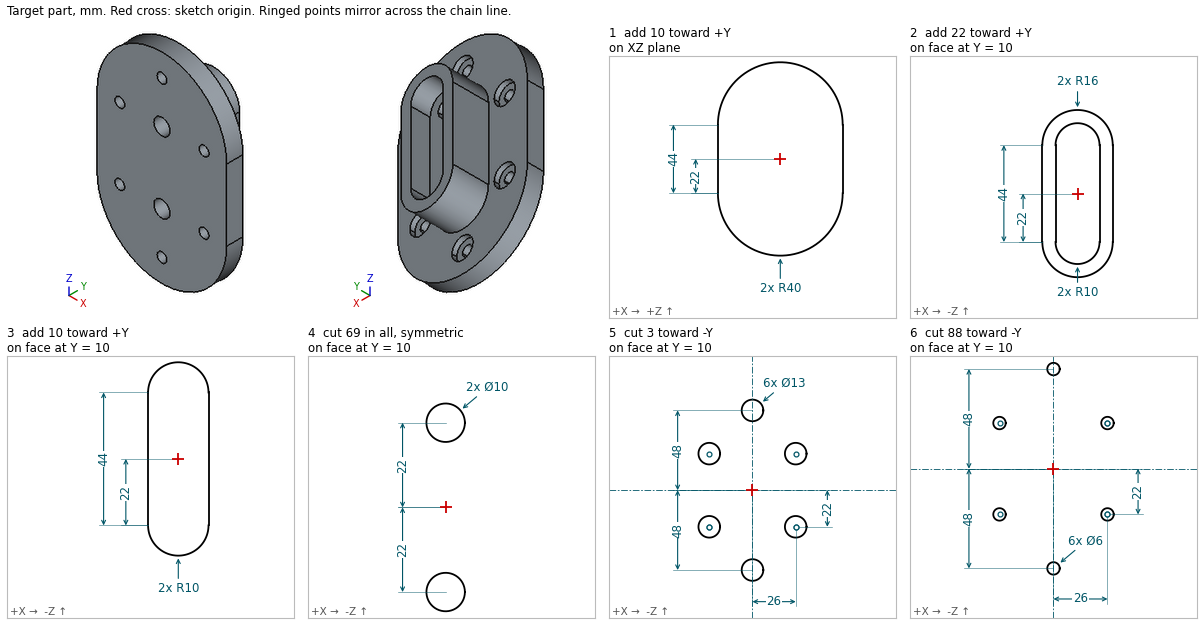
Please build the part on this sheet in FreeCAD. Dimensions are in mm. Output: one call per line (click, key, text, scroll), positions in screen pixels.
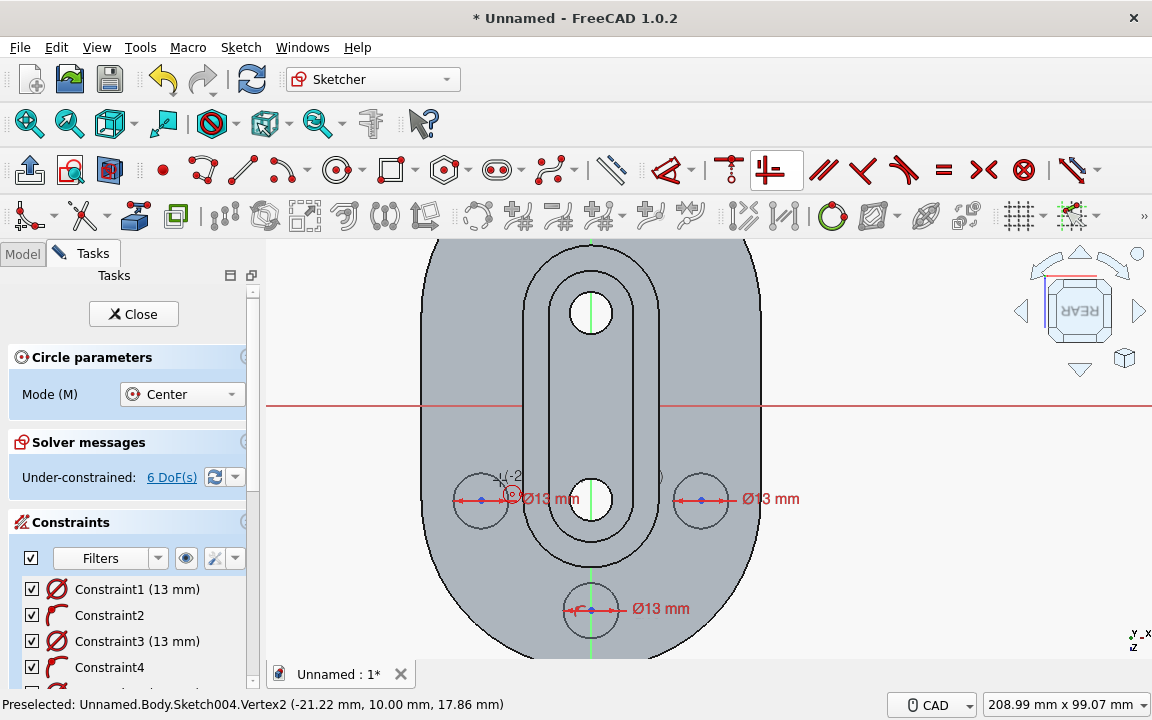
click(701, 313)
move(721, 294)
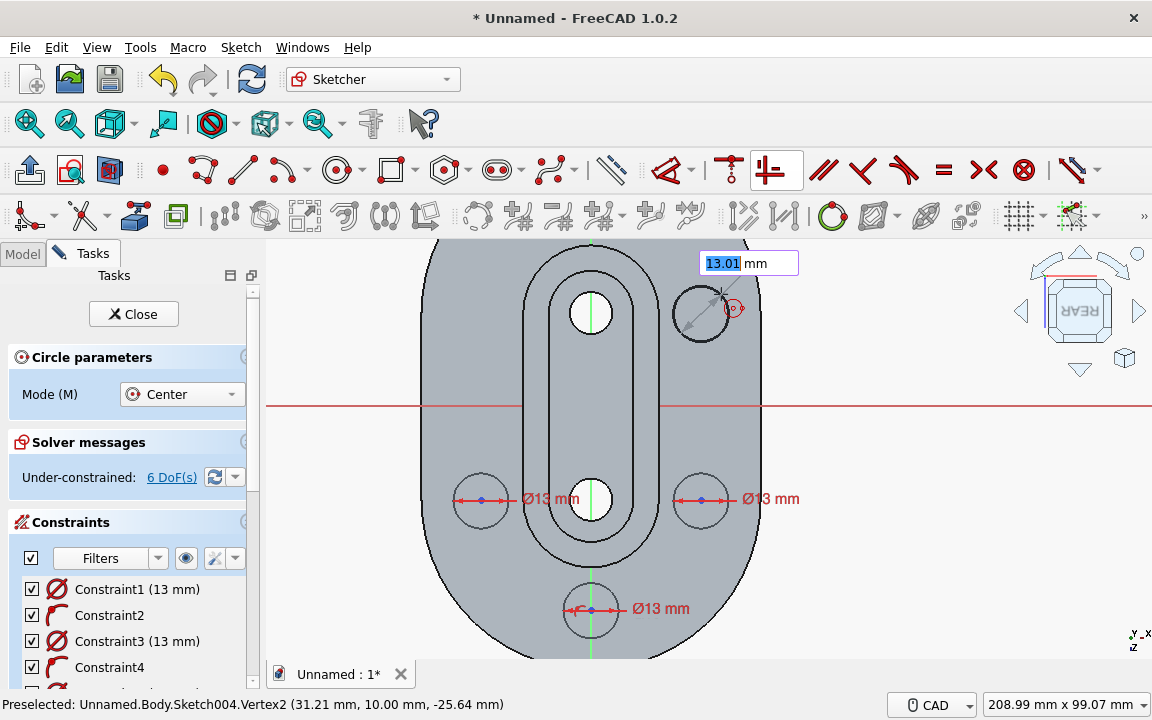
text(13)
key(Return)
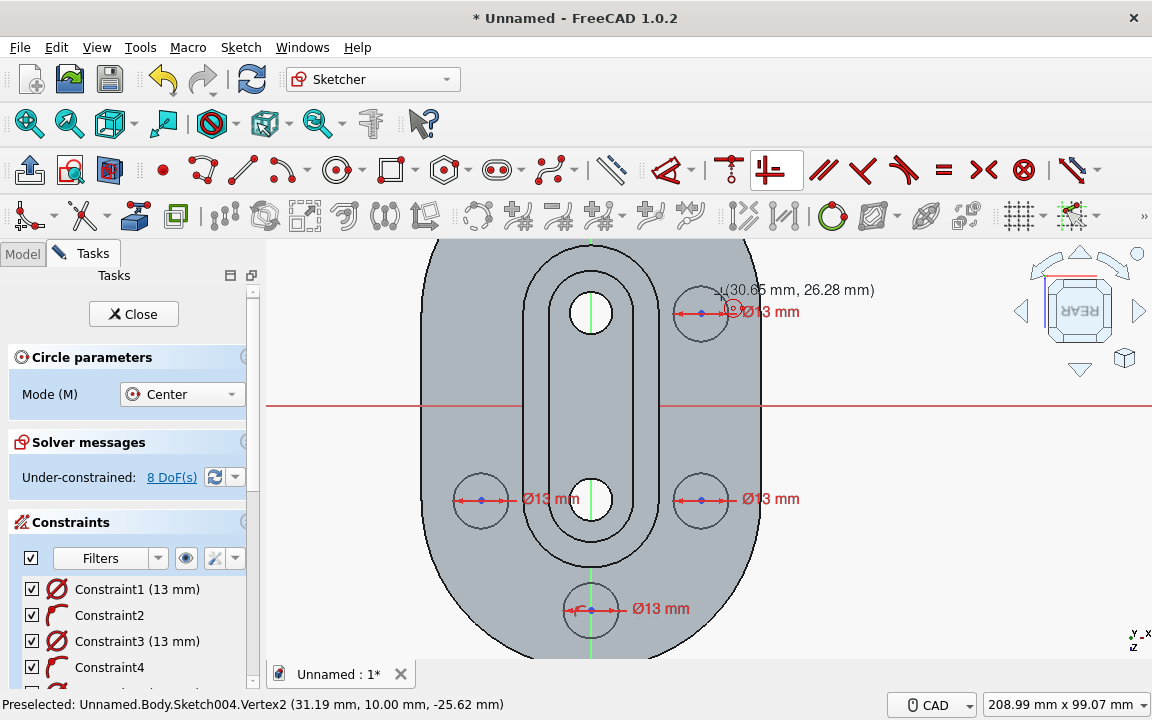
click(481, 313)
move(500, 294)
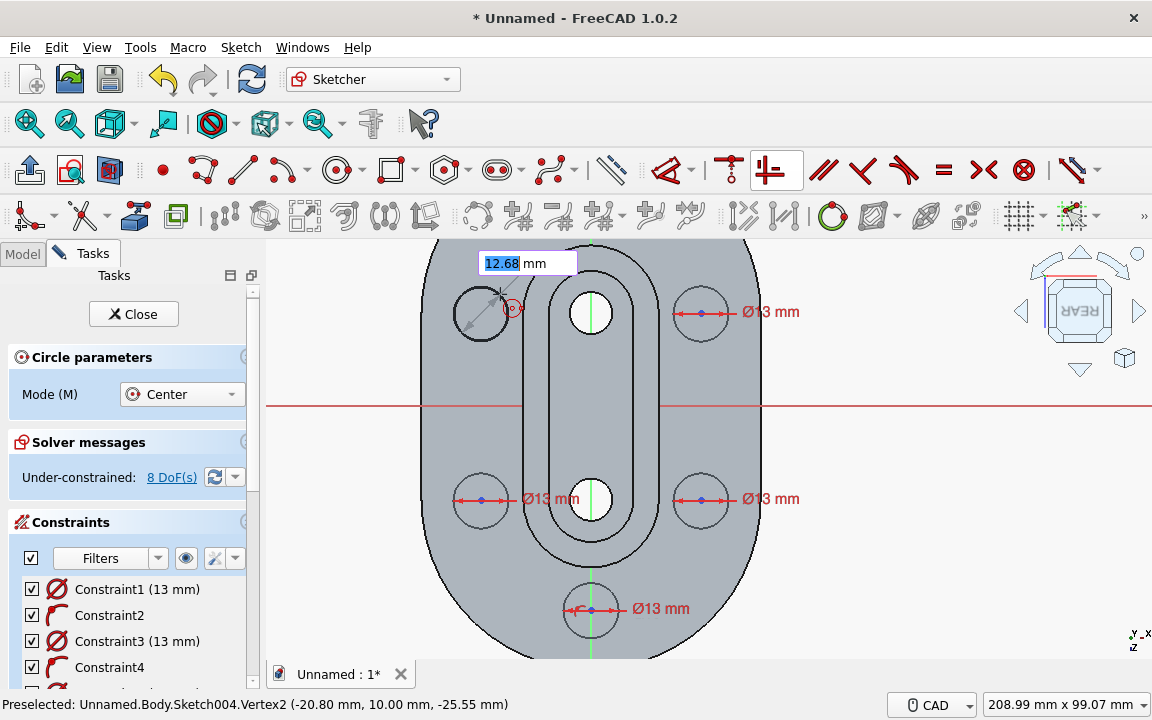
text(13)
key(Return)
key(Escape)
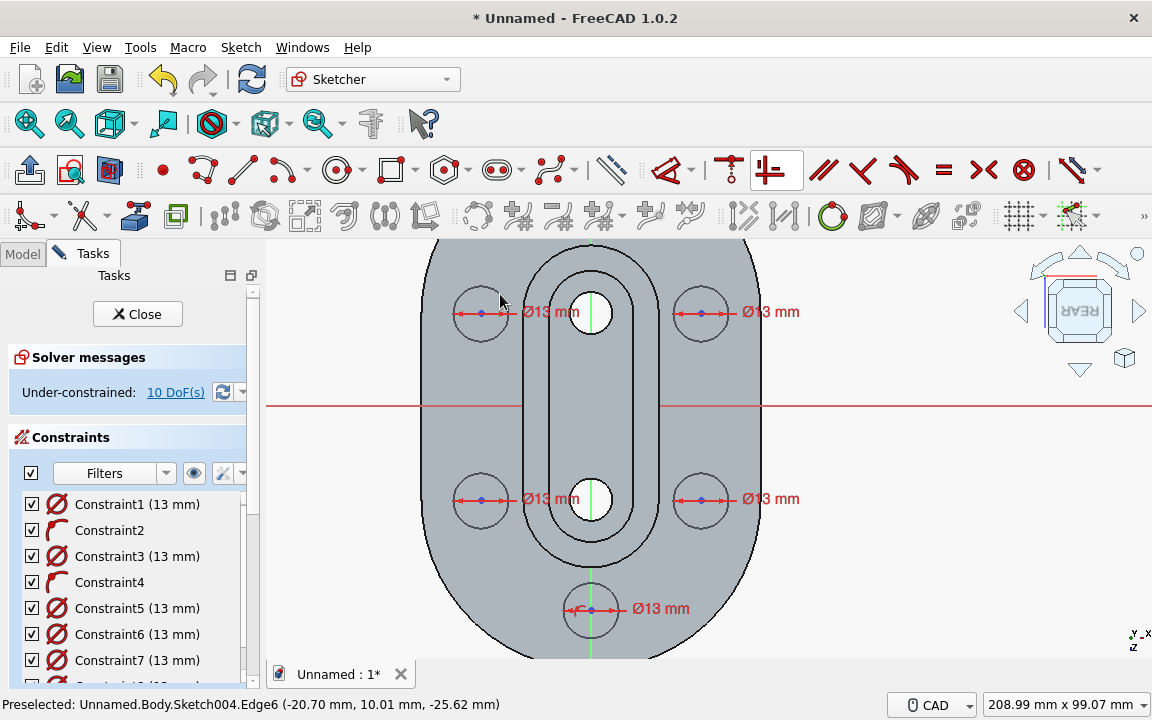
click(701, 501)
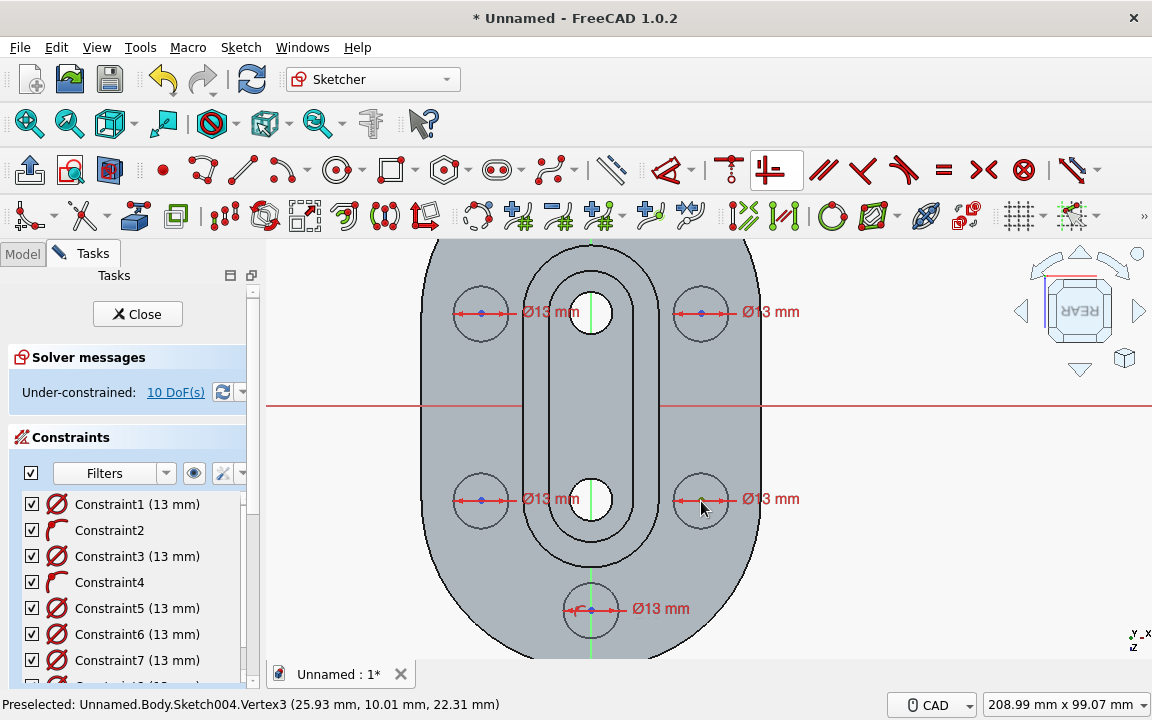
click(481, 501)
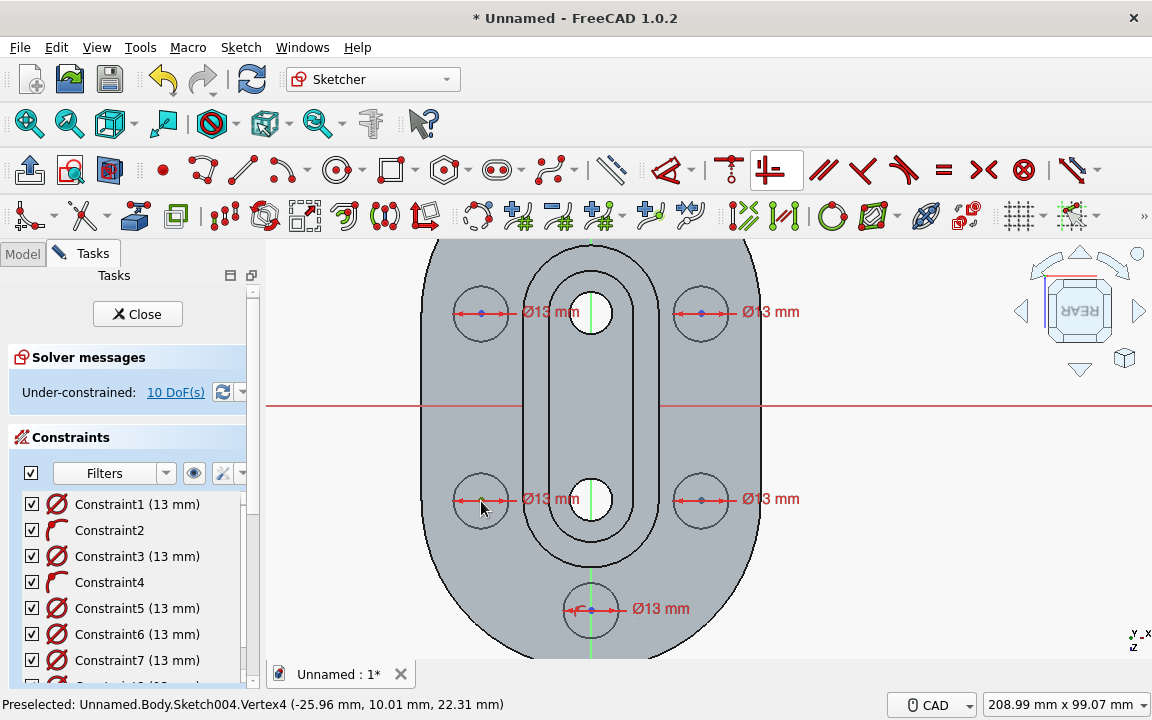
click(591, 553)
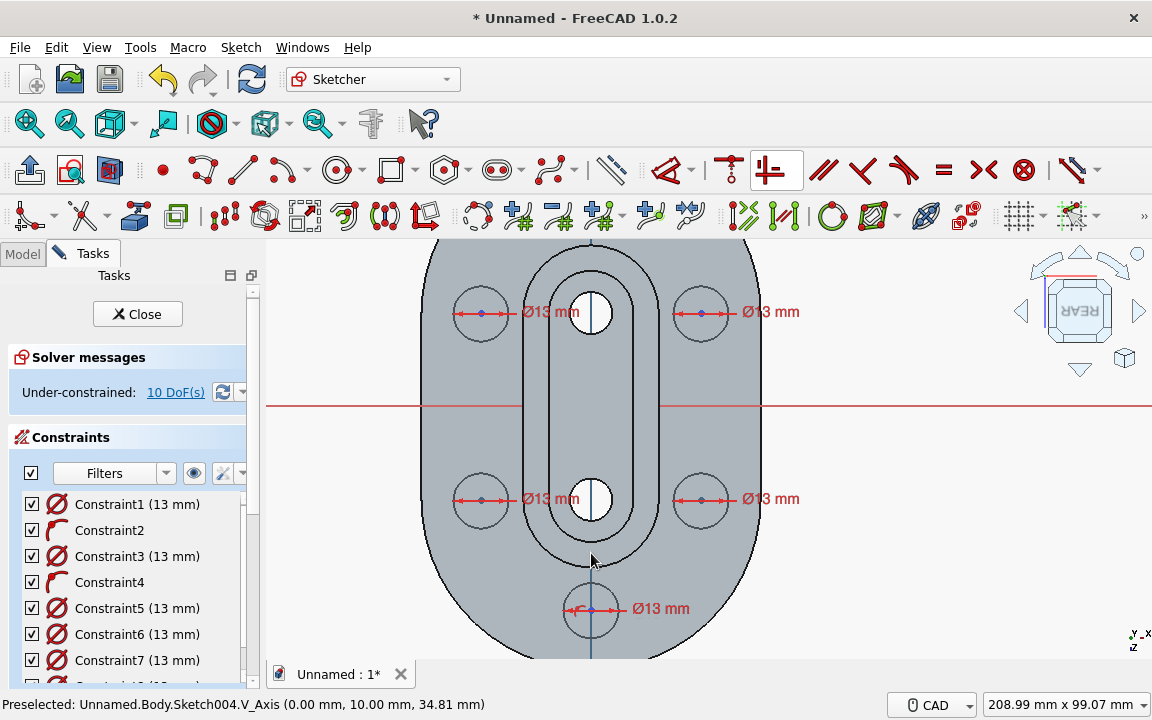
click(984, 170)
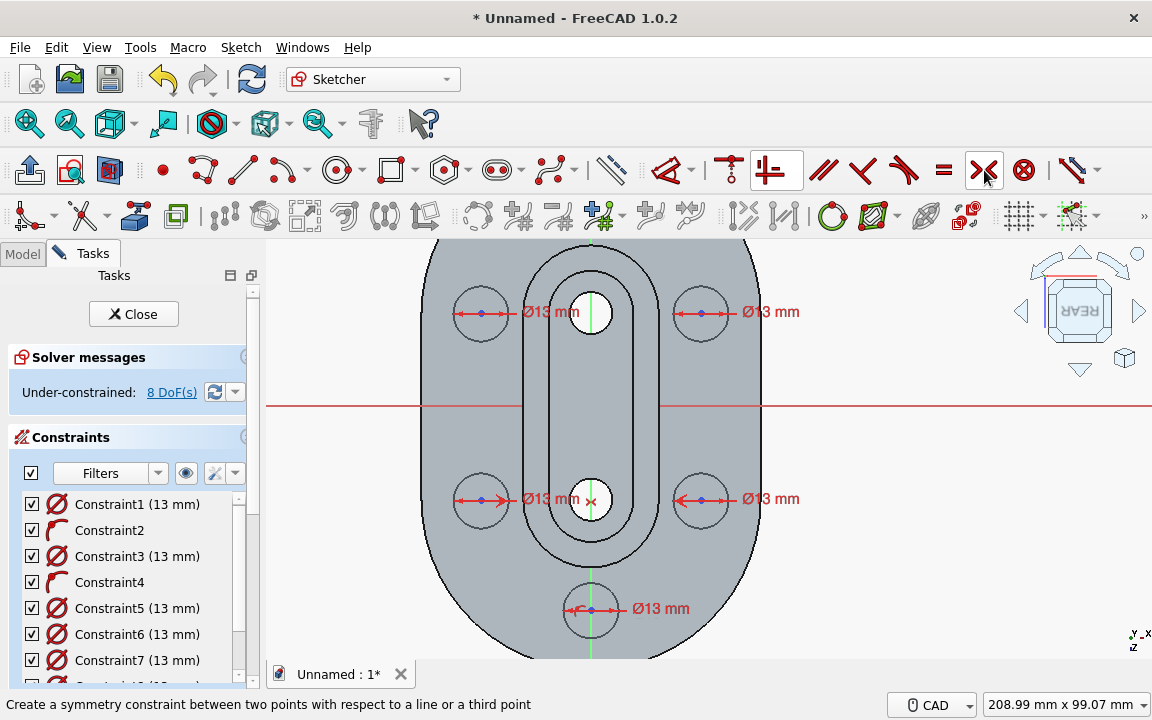
click(701, 501)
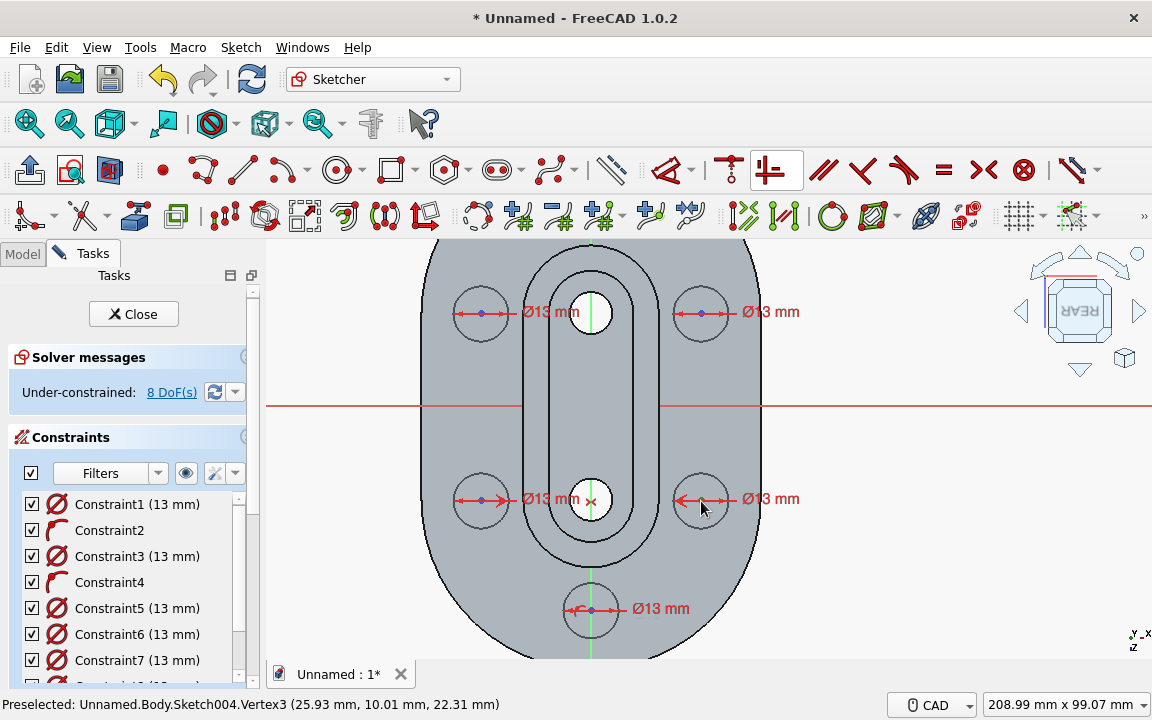
click(701, 314)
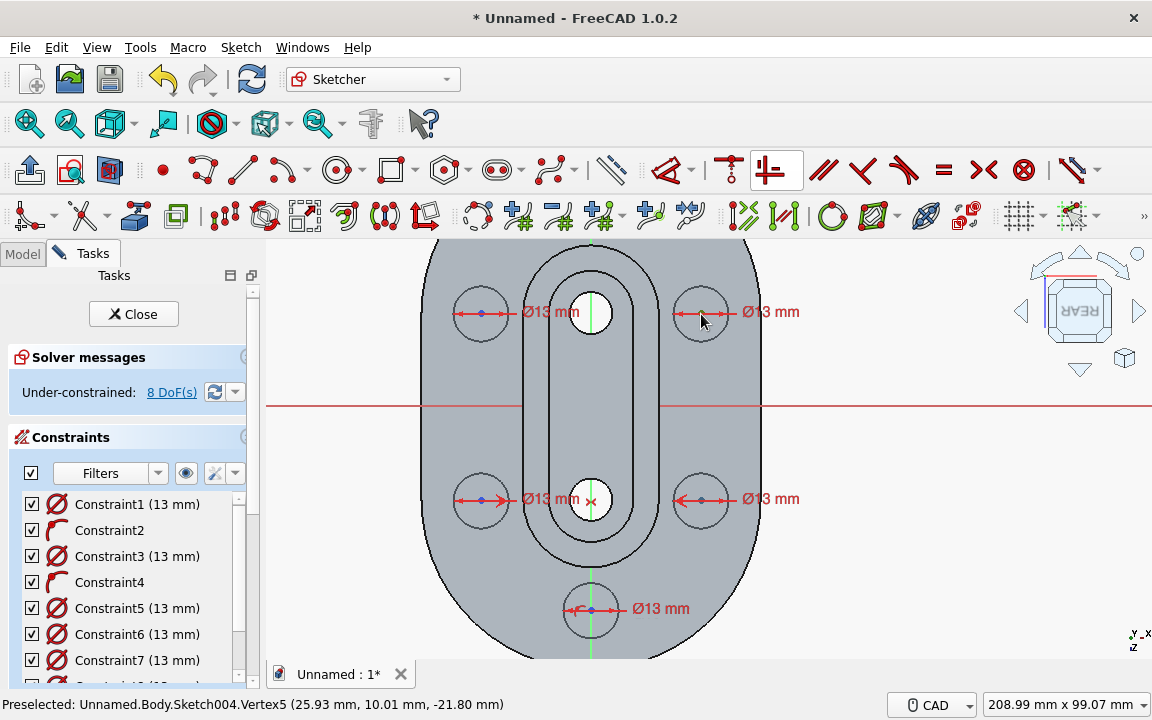
click(344, 406)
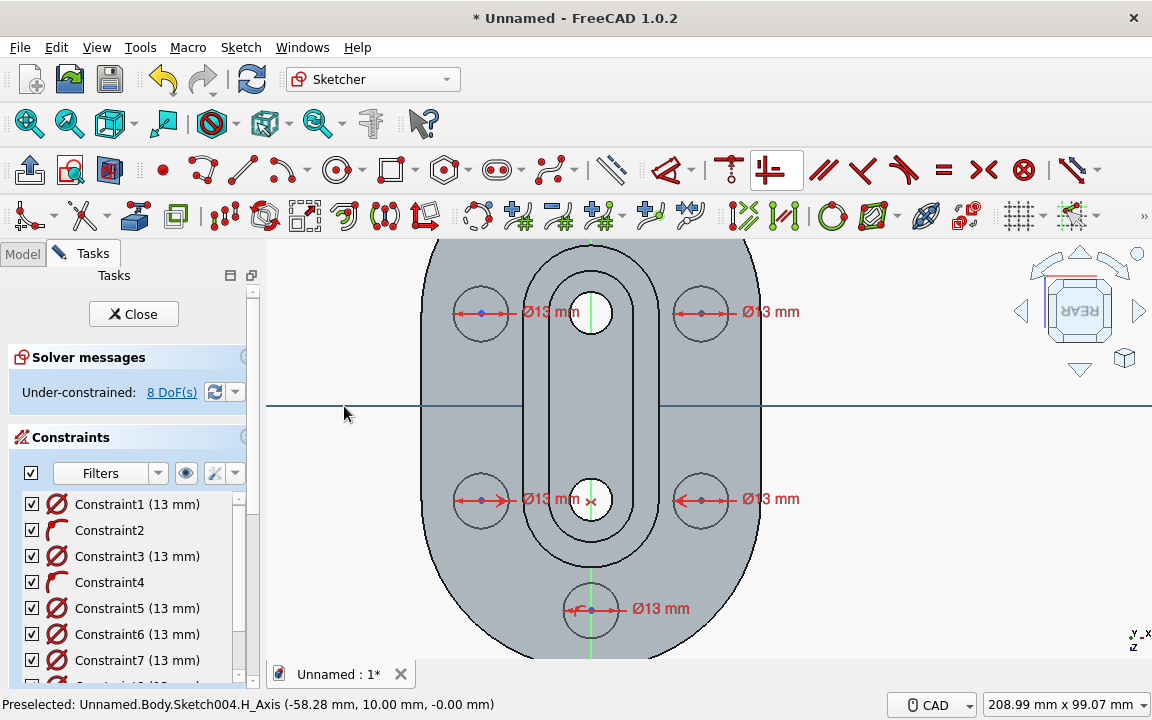
click(984, 170)